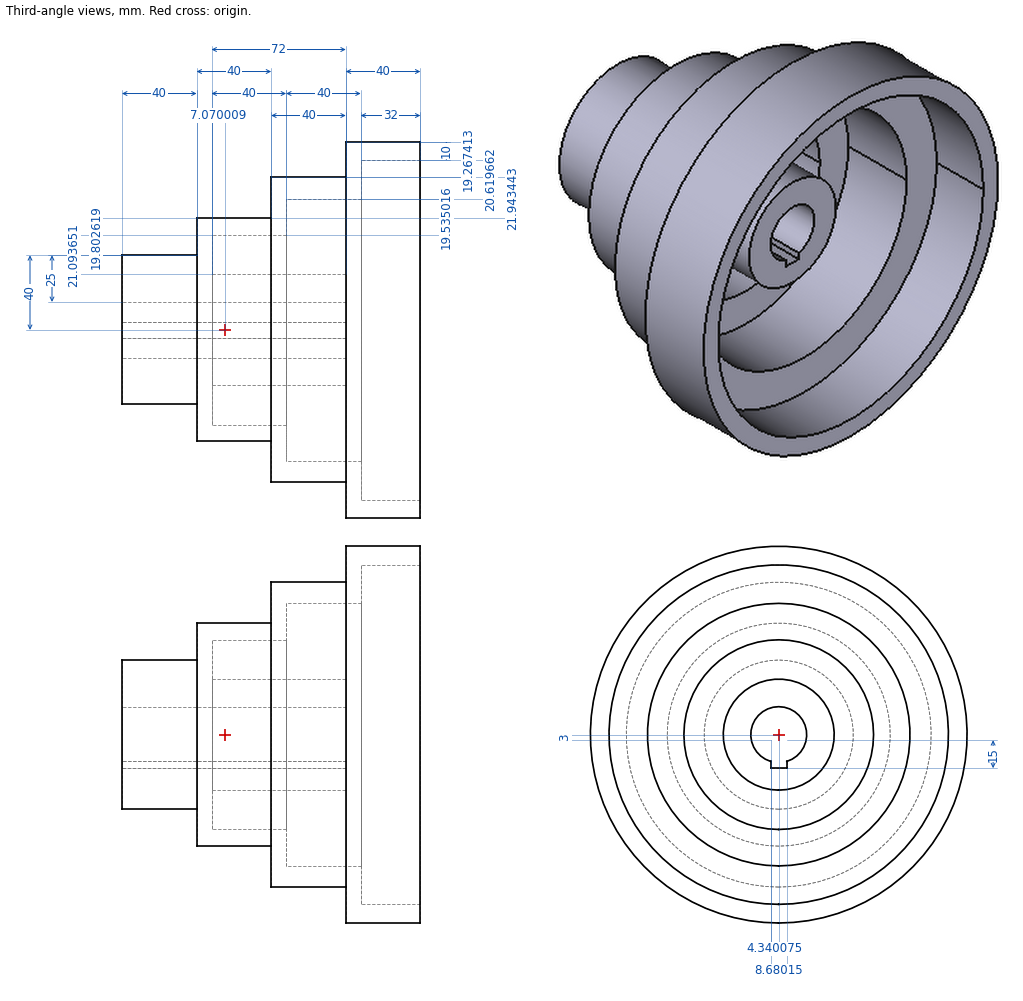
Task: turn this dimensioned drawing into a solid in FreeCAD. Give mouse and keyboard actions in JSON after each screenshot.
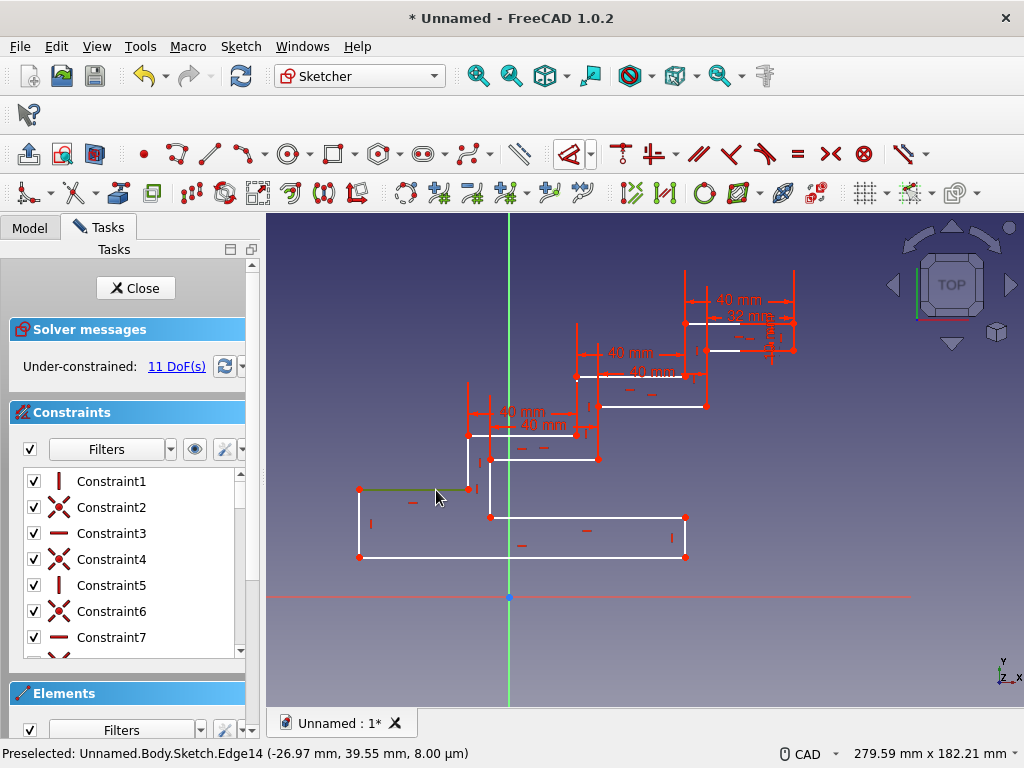
{"action": "left_click", "coordinate": [590, 154]}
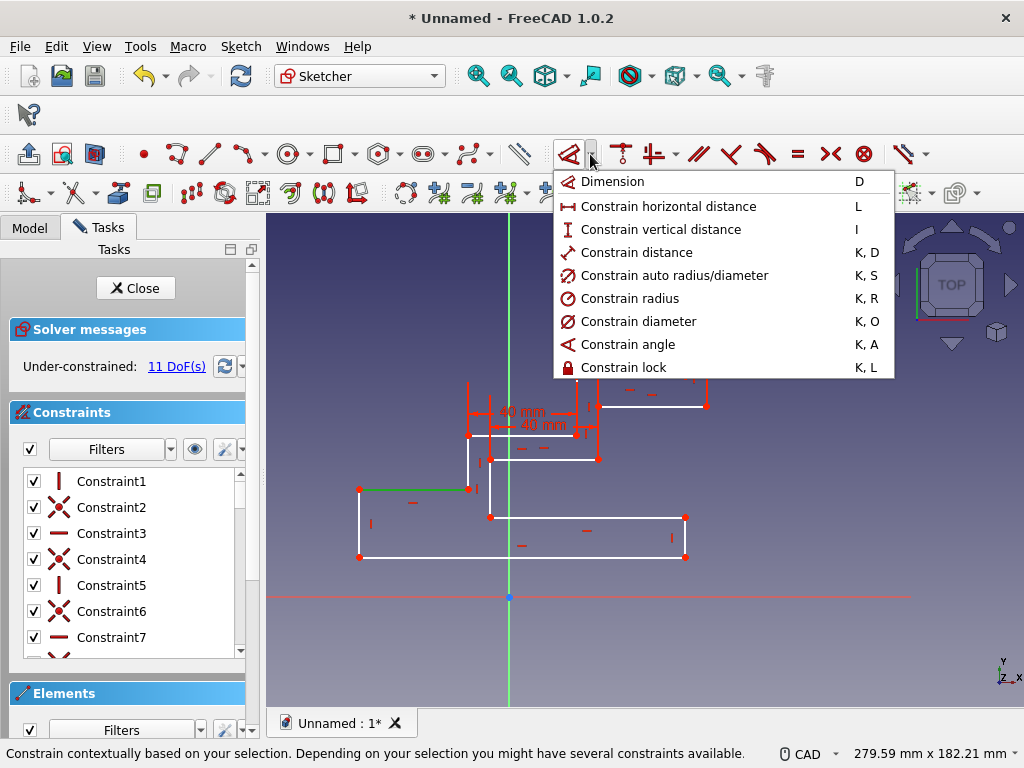
{"action": "left_click", "coordinate": [724, 206]}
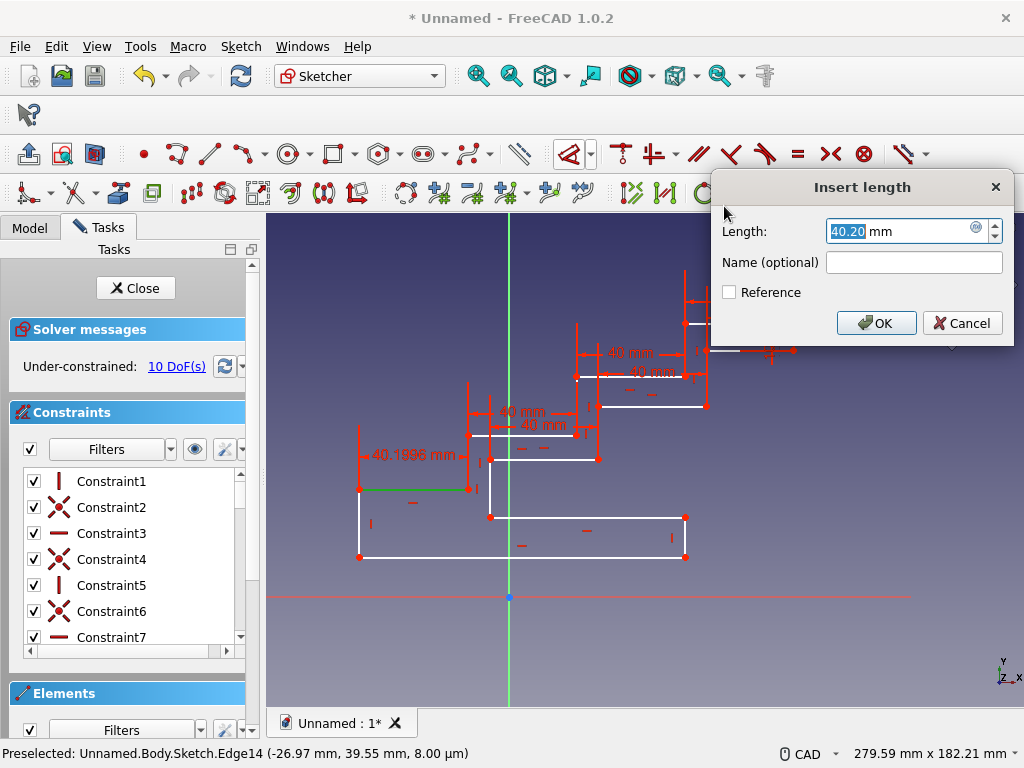
{"action": "type", "text": "40"}
{"action": "key", "text": "Return"}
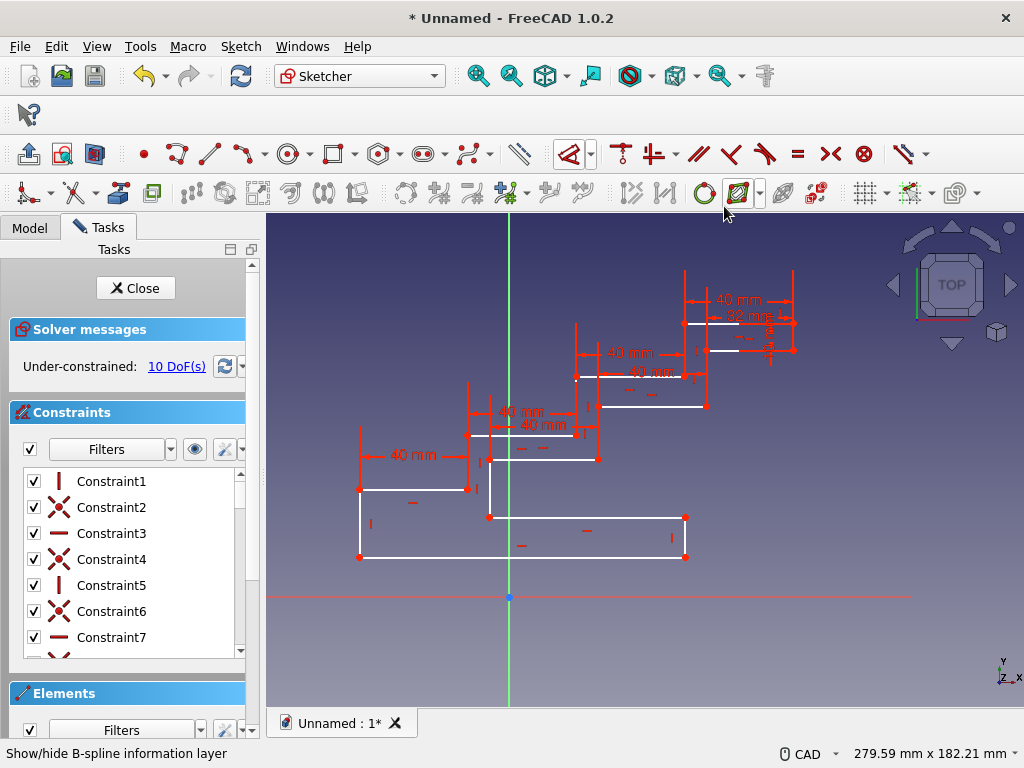
{"action": "left_click", "coordinate": [360, 510]}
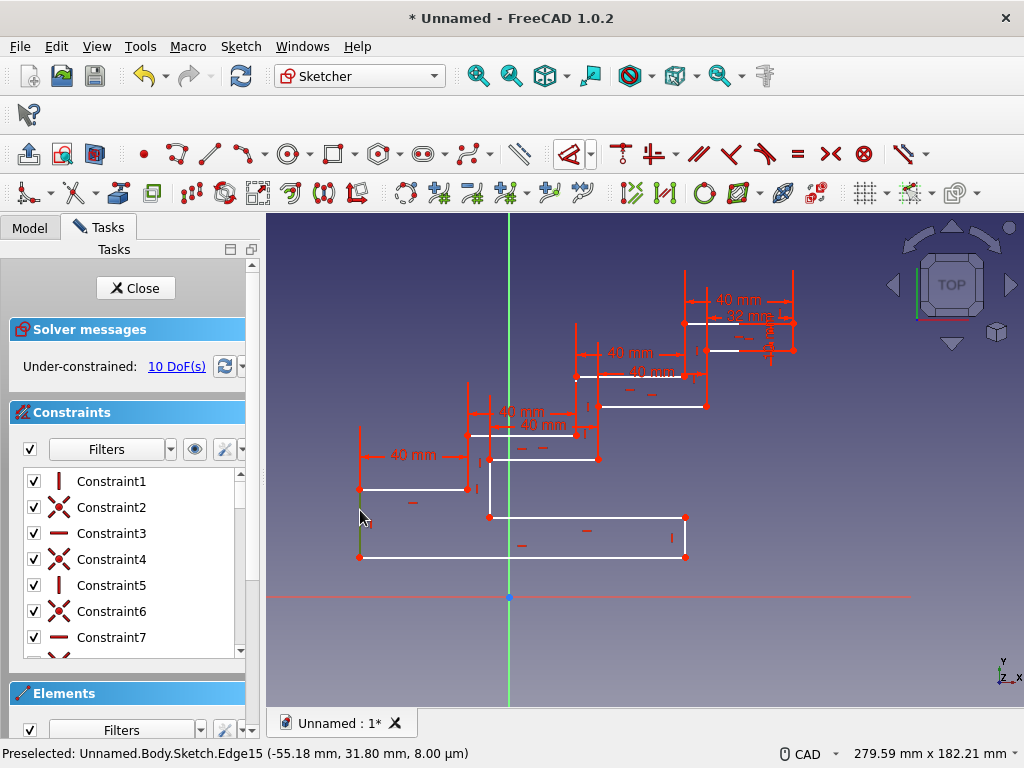
{"action": "left_click", "coordinate": [590, 154]}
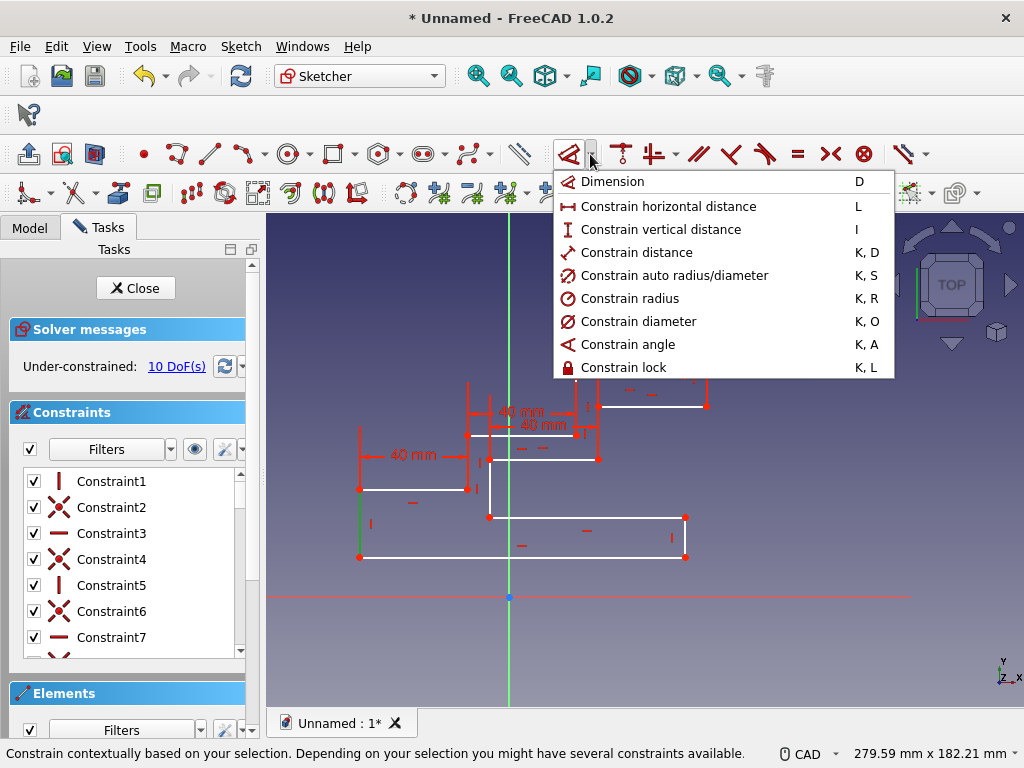
{"action": "left_click", "coordinate": [724, 230]}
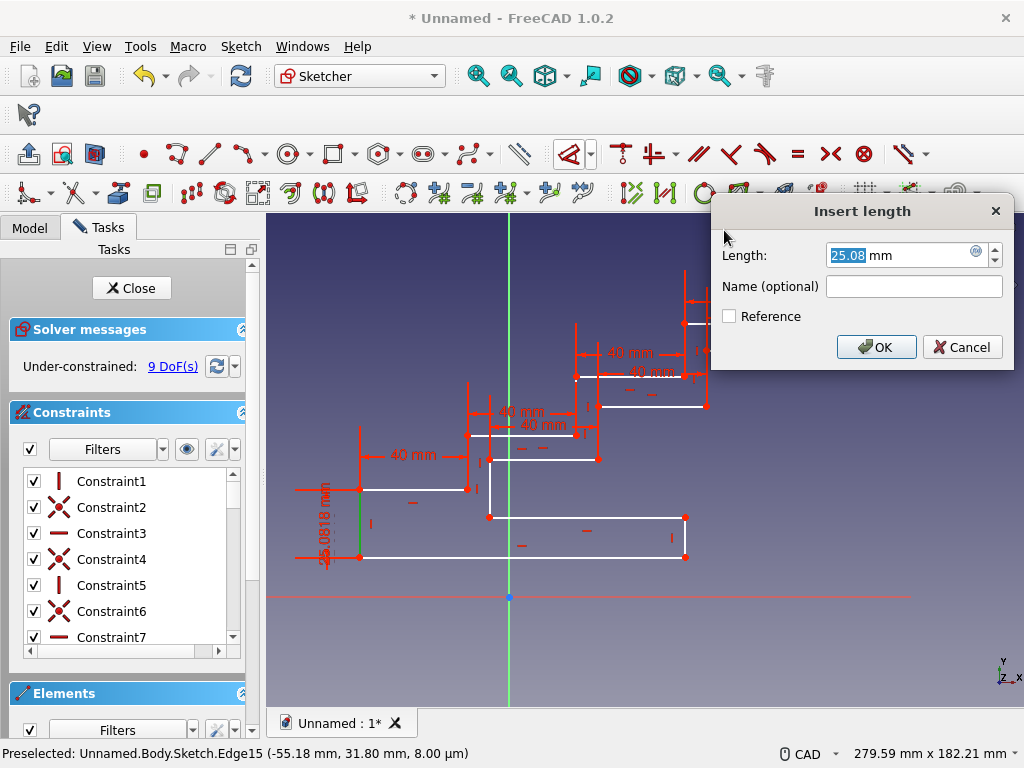
{"action": "type", "text": "25"}
{"action": "key", "text": "Return"}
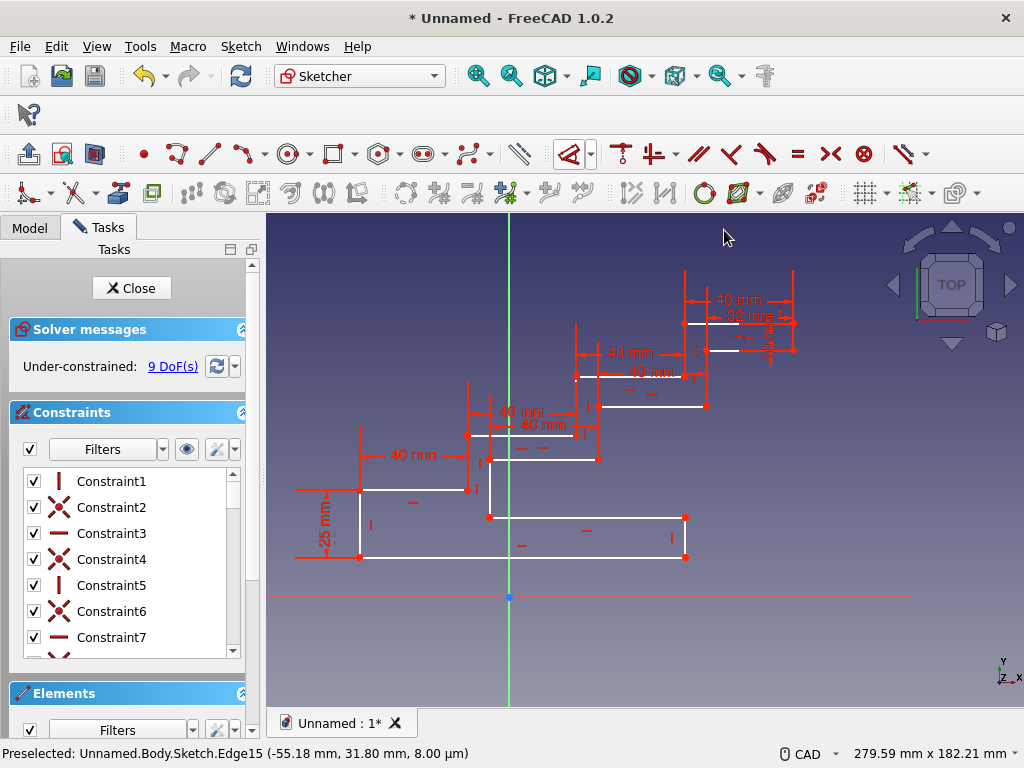
{"action": "left_click", "coordinate": [627, 518]}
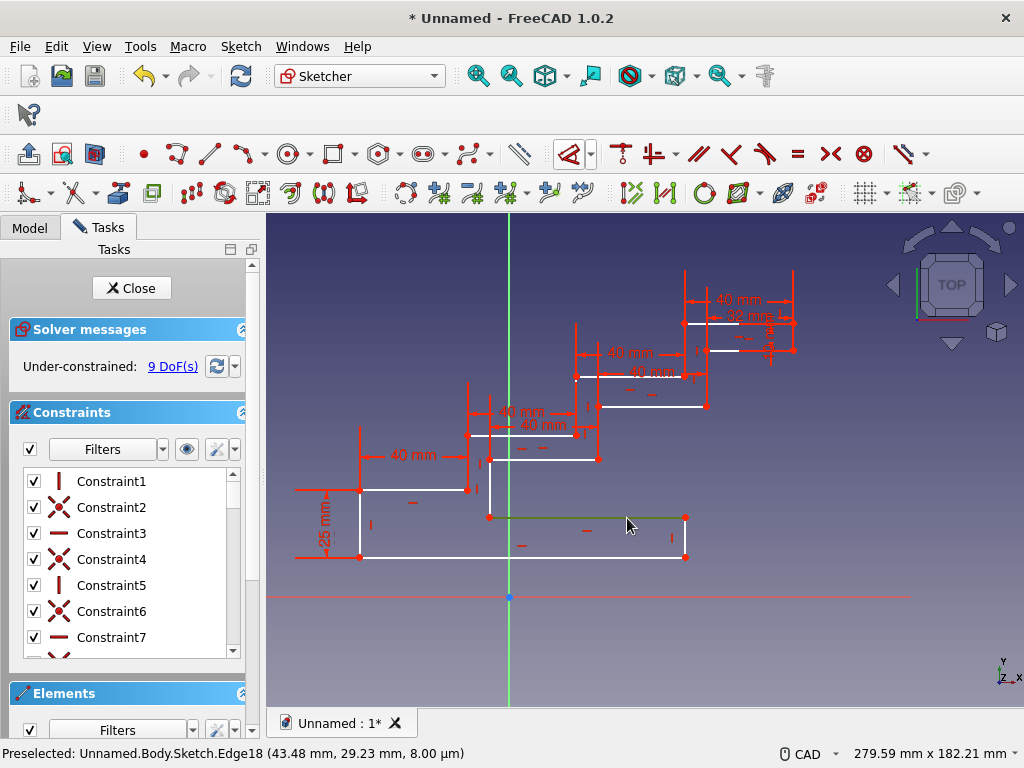
{"action": "left_click", "coordinate": [590, 154]}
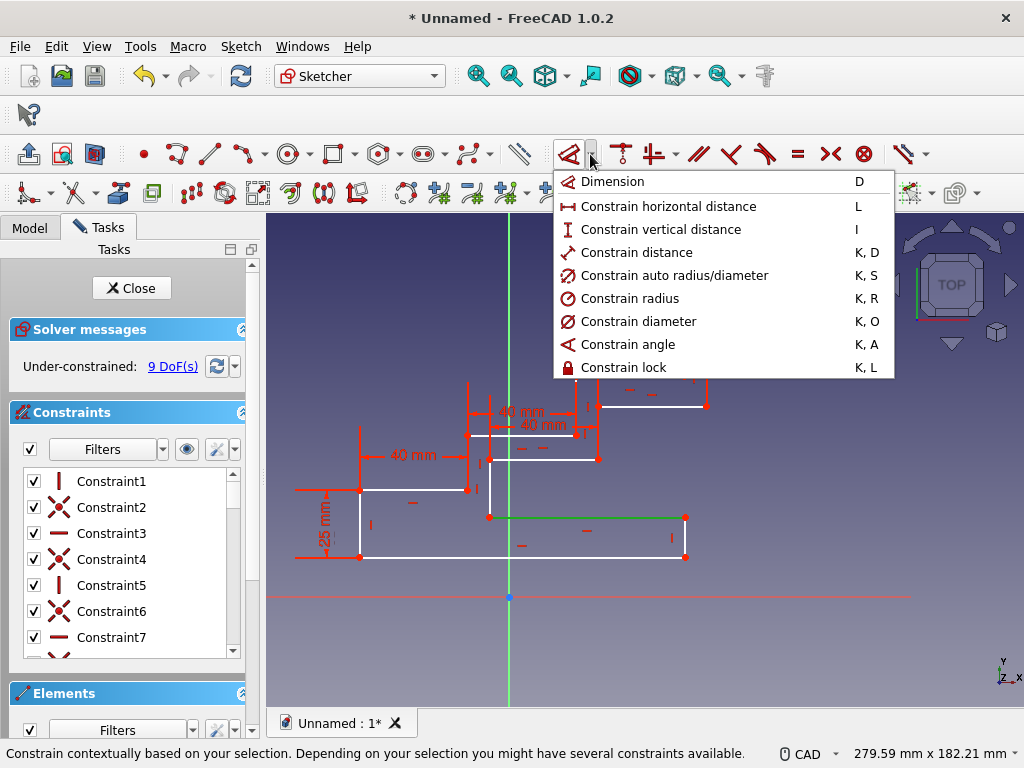
{"action": "left_click", "coordinate": [724, 206]}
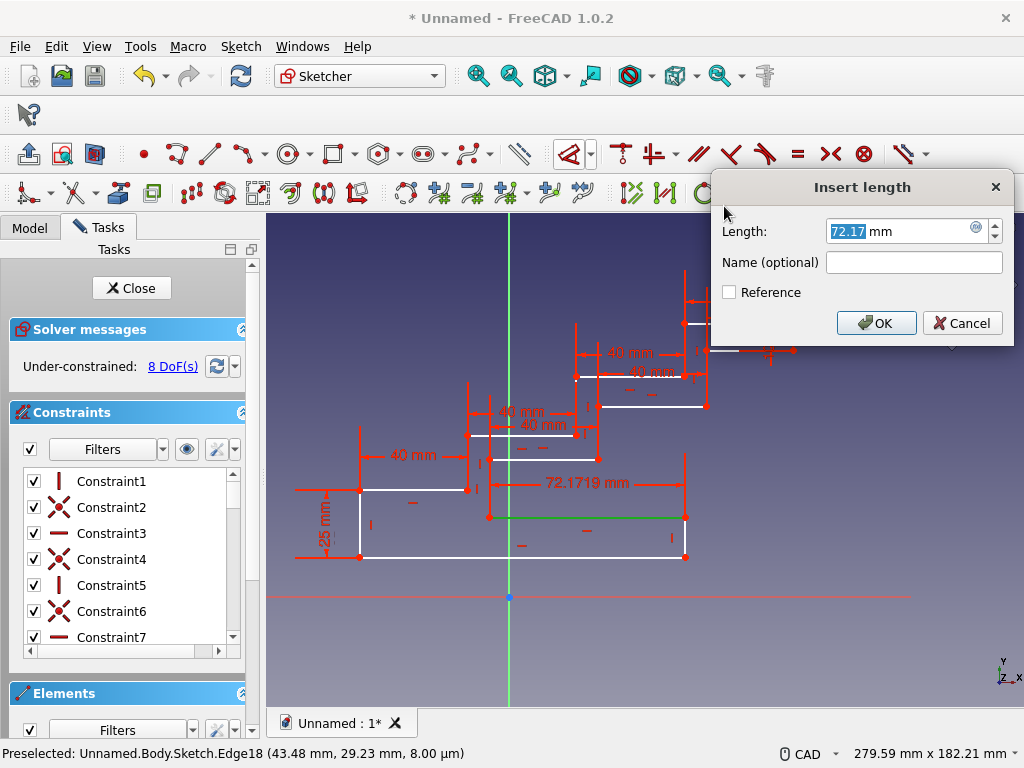
{"action": "type", "text": "72"}
{"action": "key", "text": "Return"}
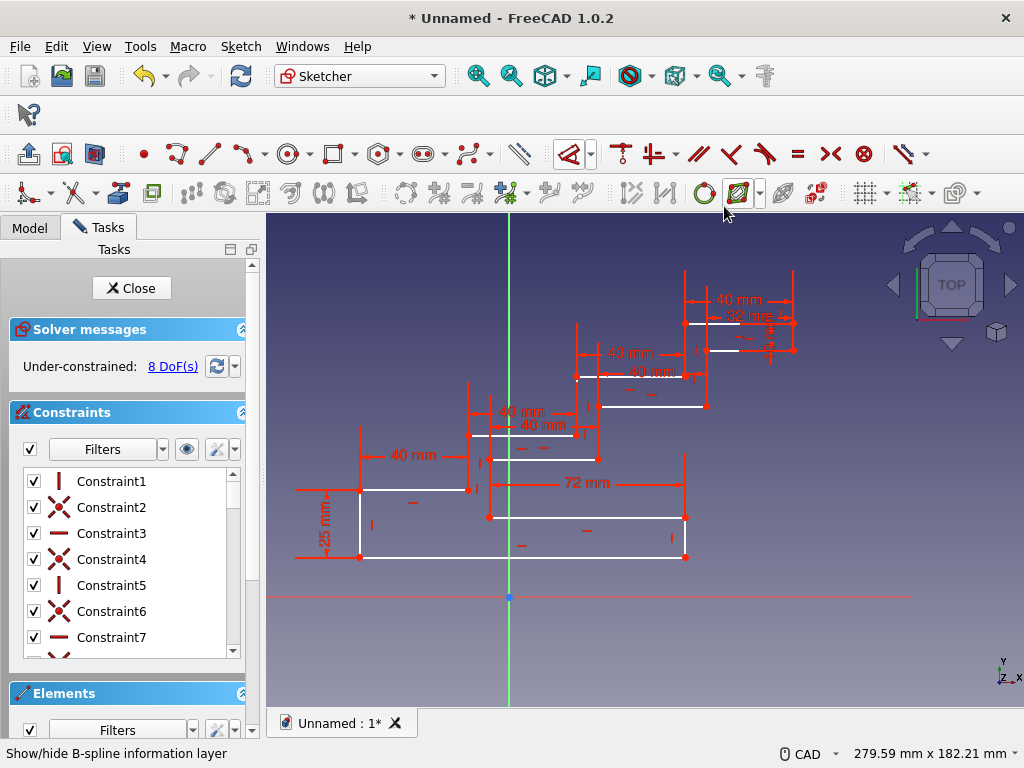
{"action": "left_click", "coordinate": [468, 490]}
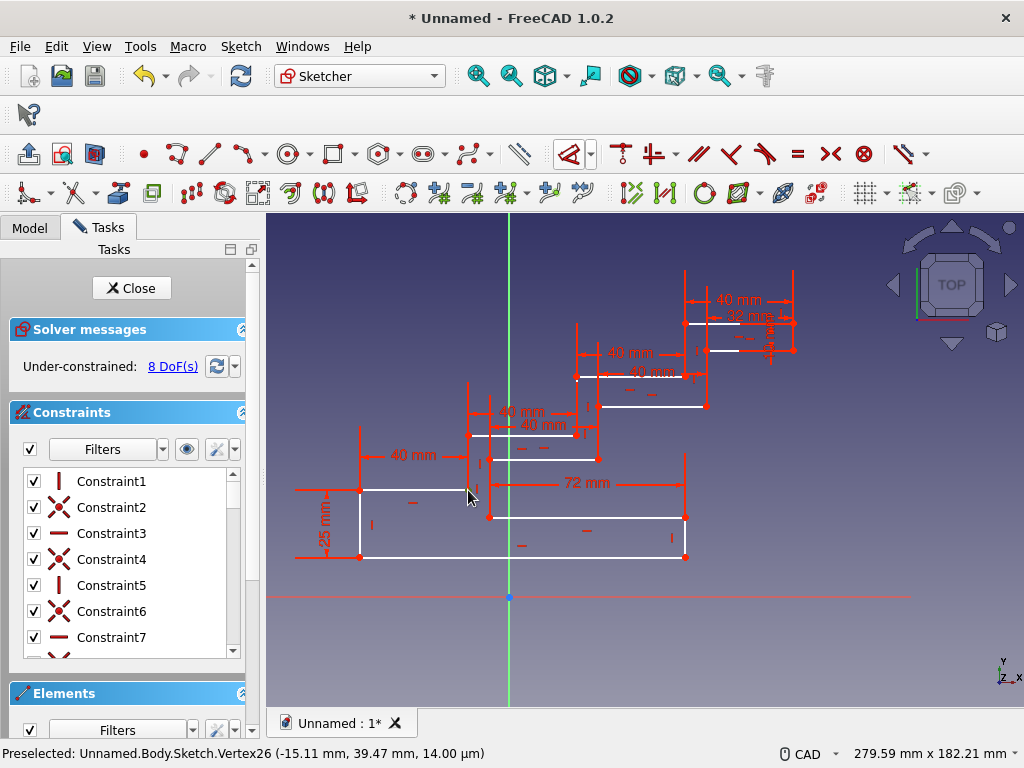
{"action": "key", "text": "i"}